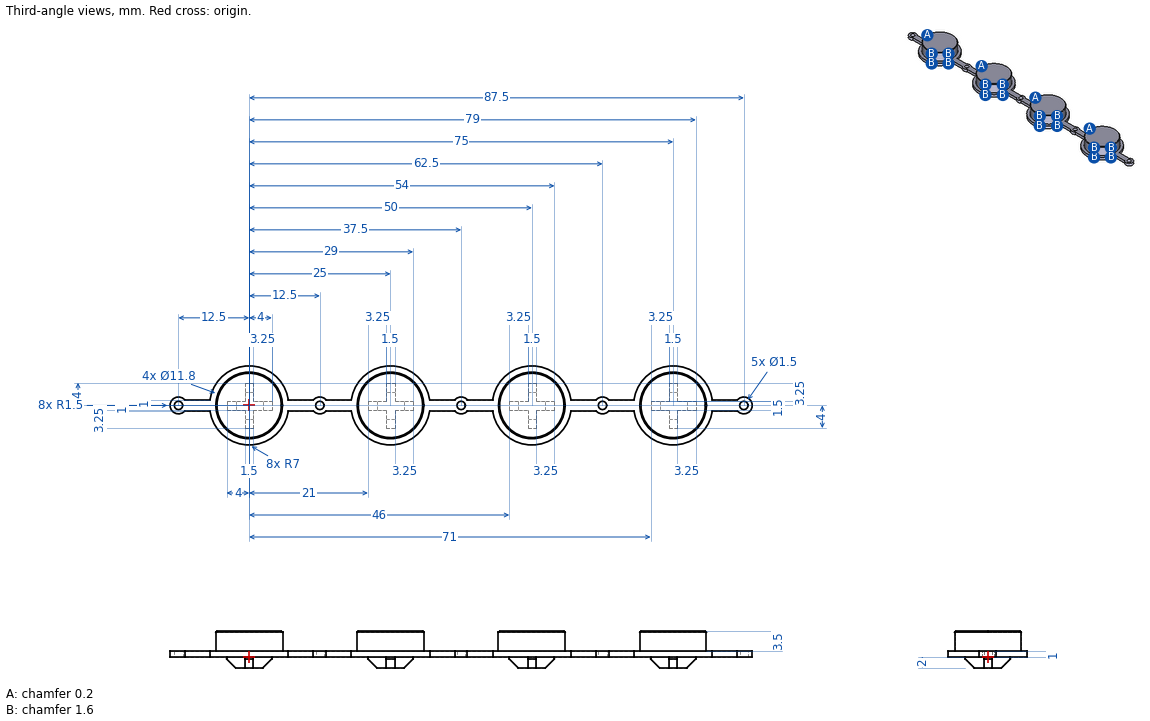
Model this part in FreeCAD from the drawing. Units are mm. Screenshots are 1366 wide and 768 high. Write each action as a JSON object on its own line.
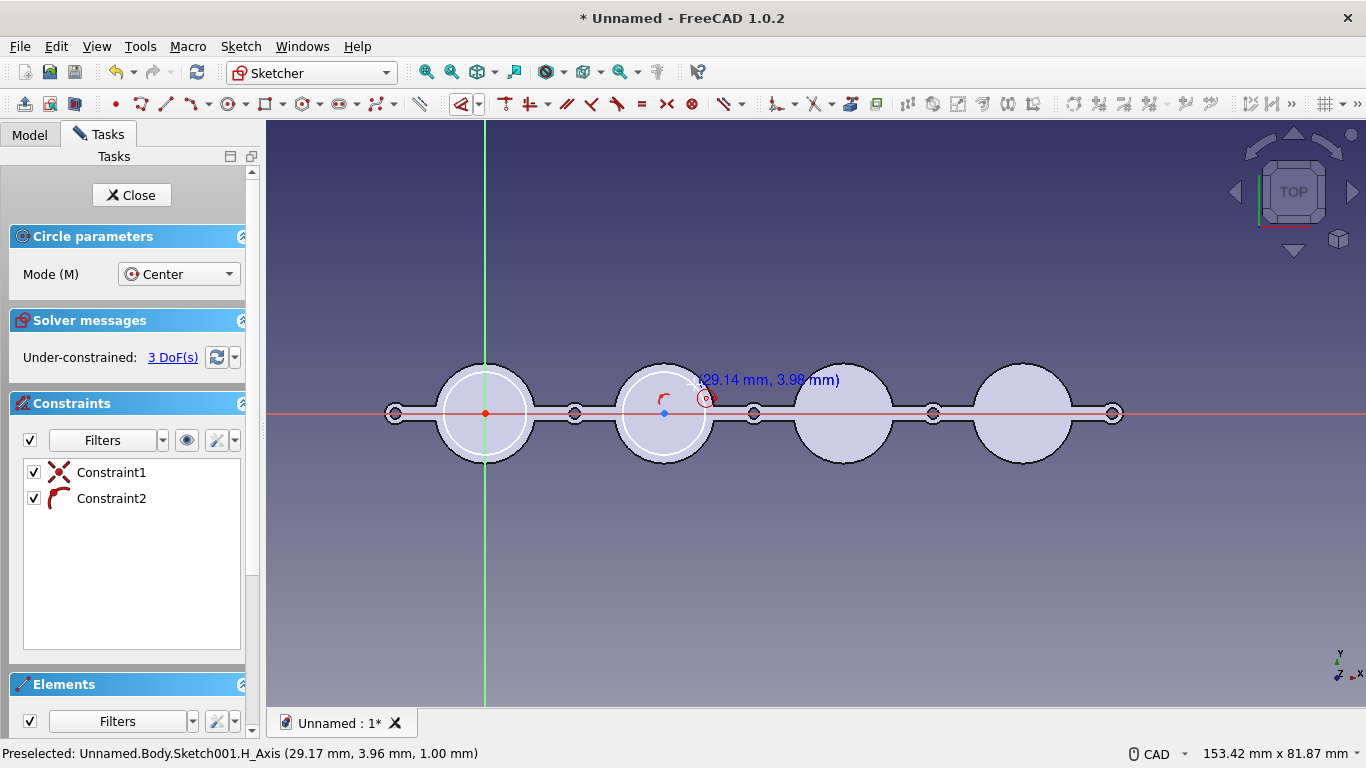
{"action": "left_click", "coordinate": [844, 414]}
{"action": "left_click", "coordinate": [873, 384]}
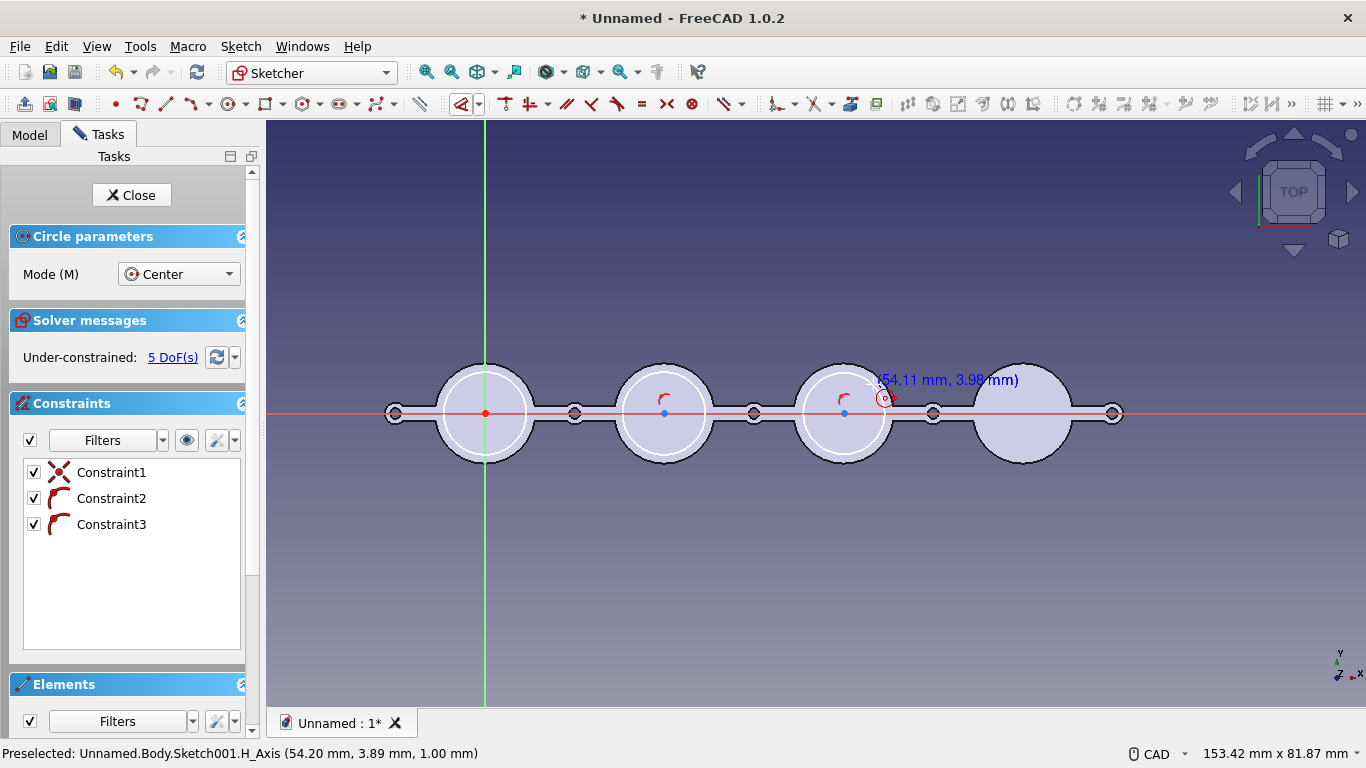
{"action": "left_click", "coordinate": [1023, 414]}
{"action": "left_click", "coordinate": [1053, 384]}
{"action": "key", "text": "Escape"}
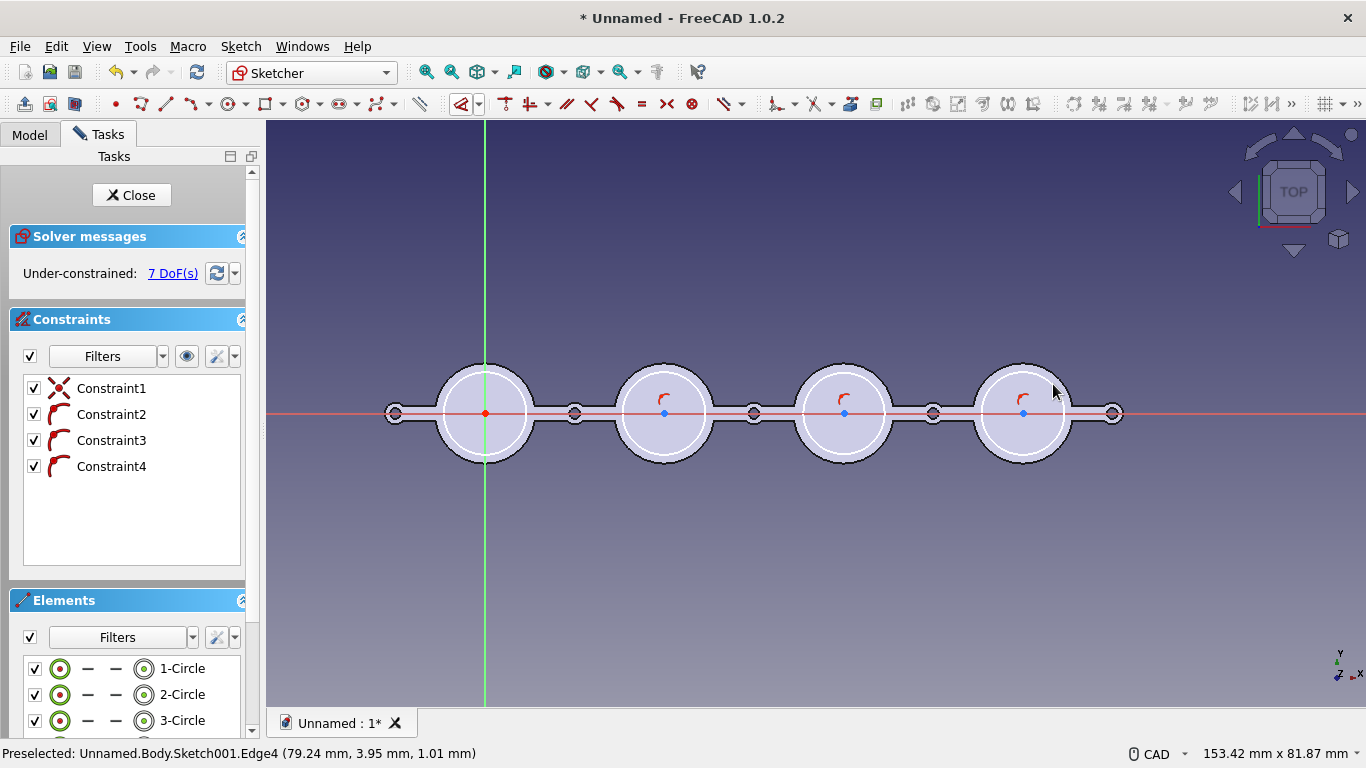
{"action": "left_click", "coordinate": [514, 384]}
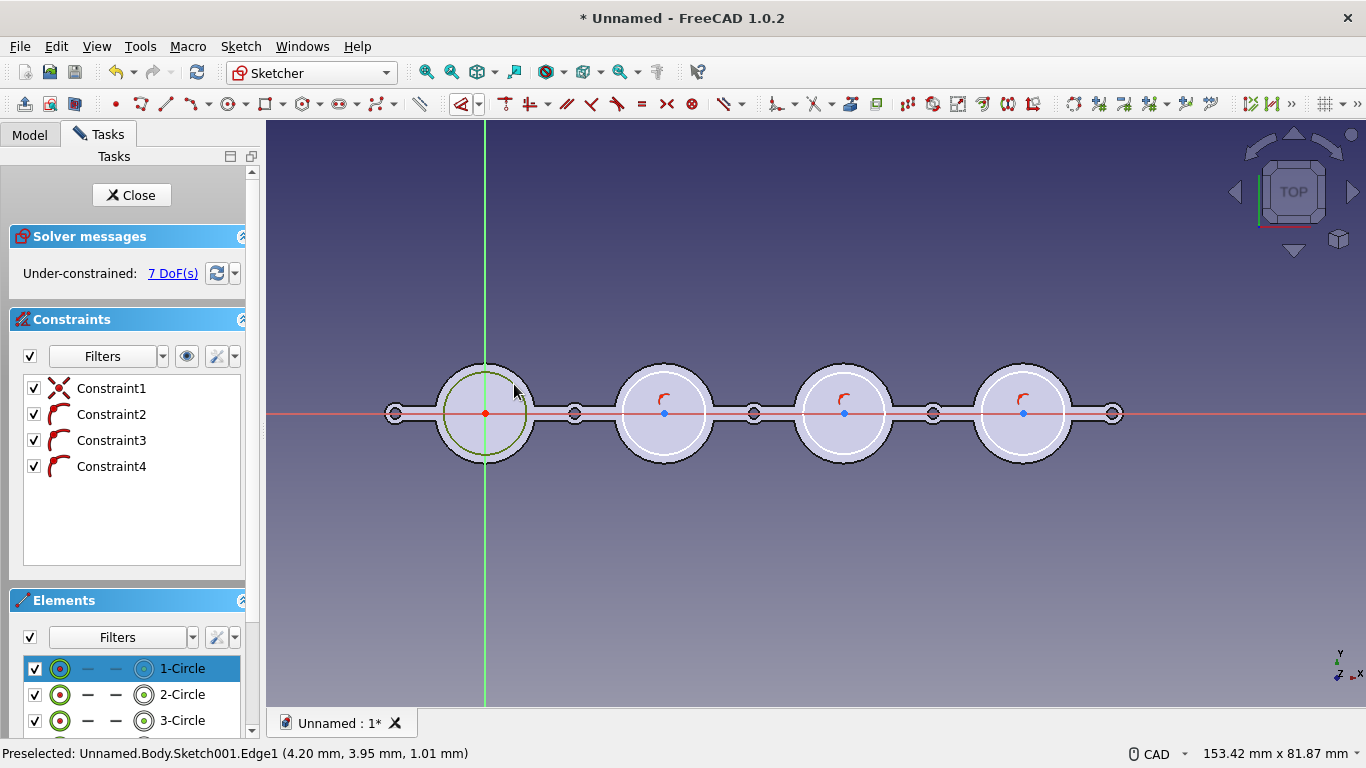
{"action": "left_click", "coordinate": [693, 384]}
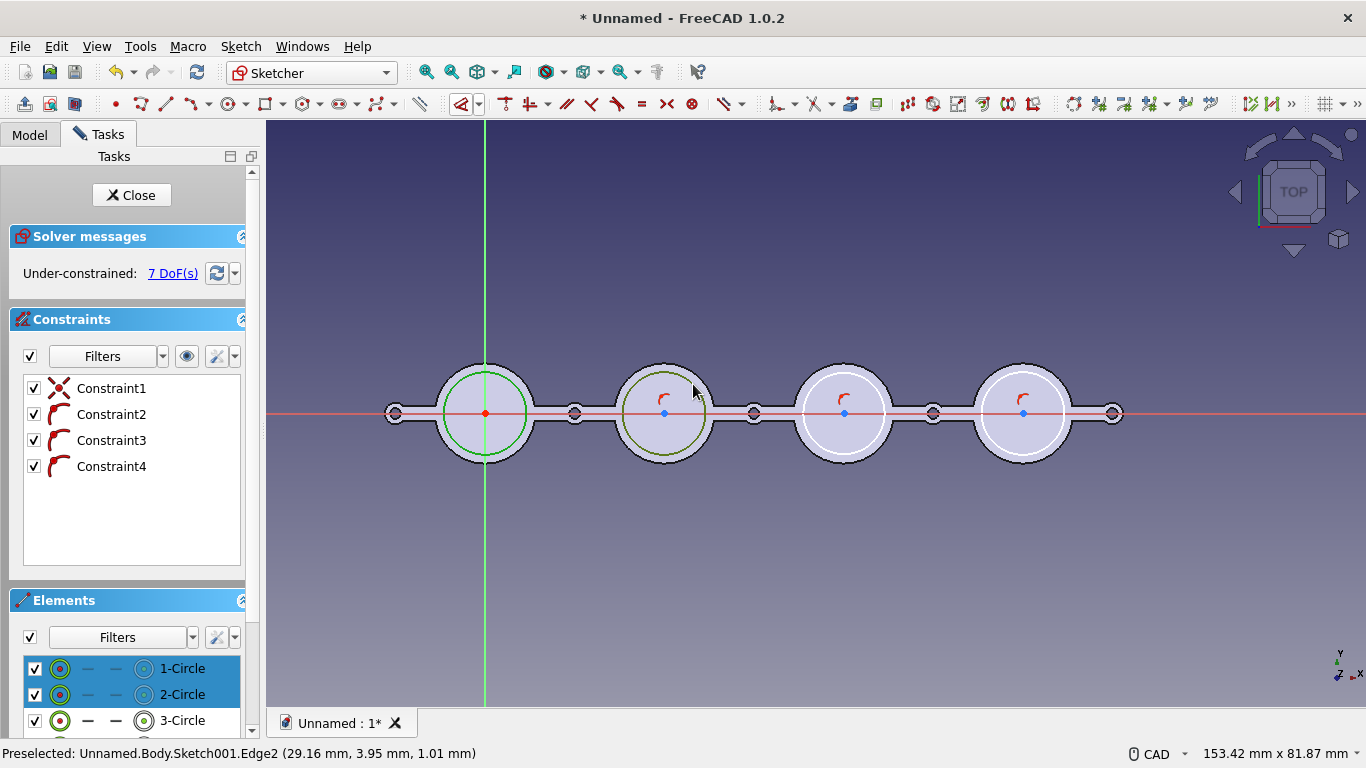
{"action": "left_click", "coordinate": [873, 385]}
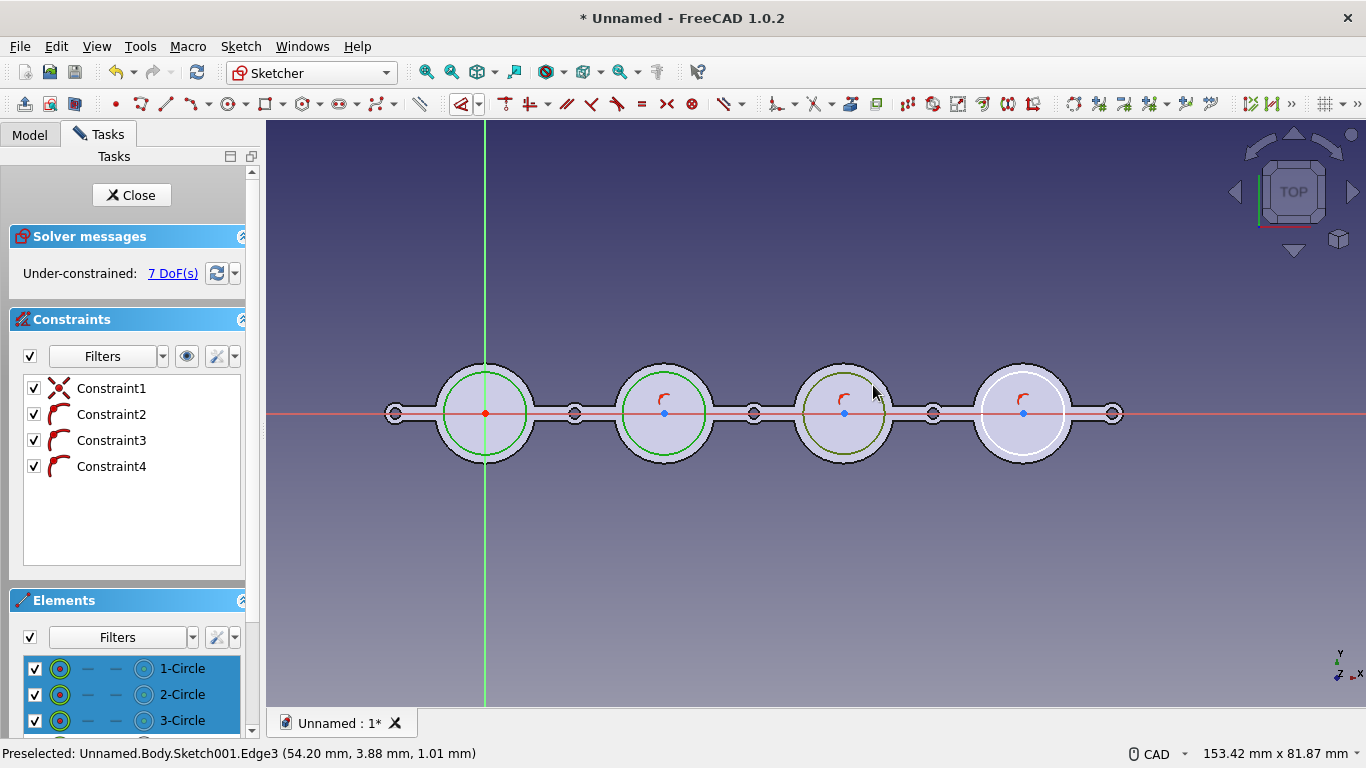
{"action": "left_click", "coordinate": [1052, 384]}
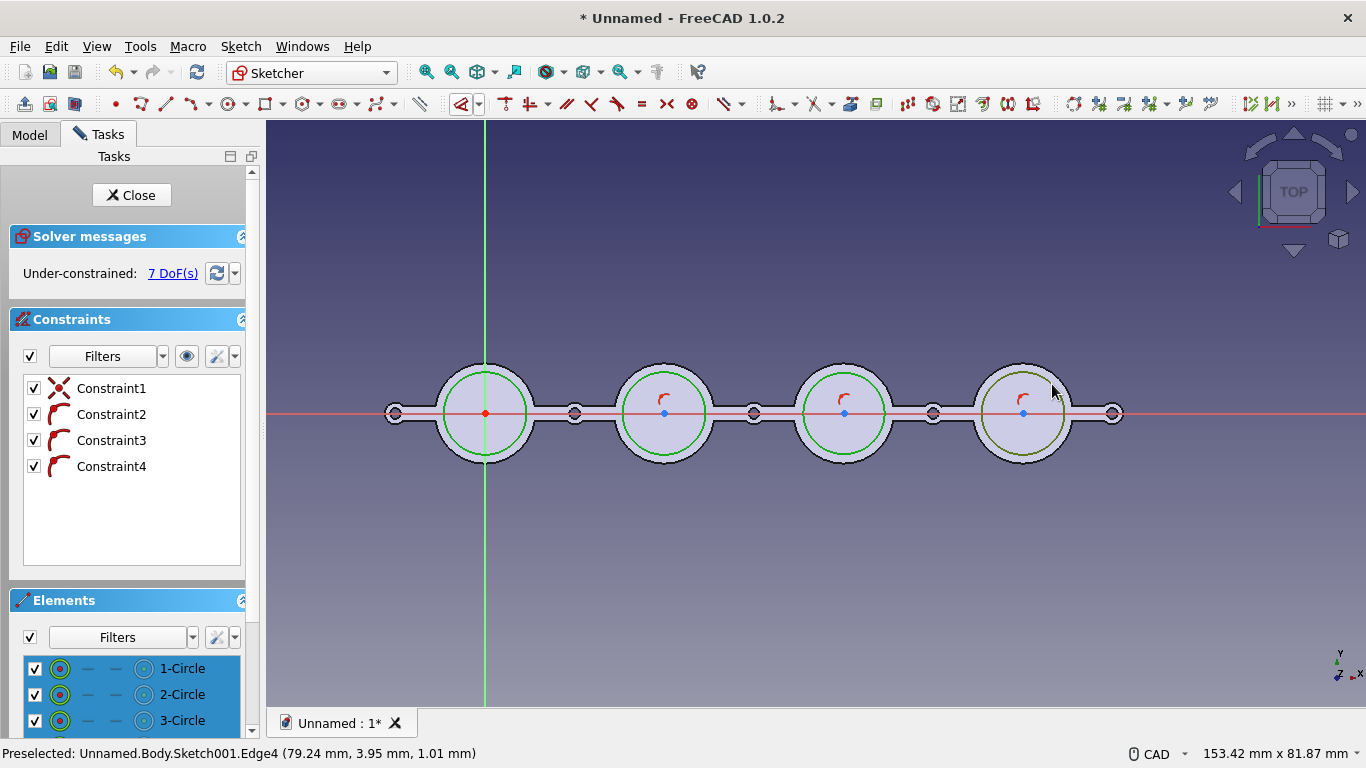
{"action": "key", "text": "e"}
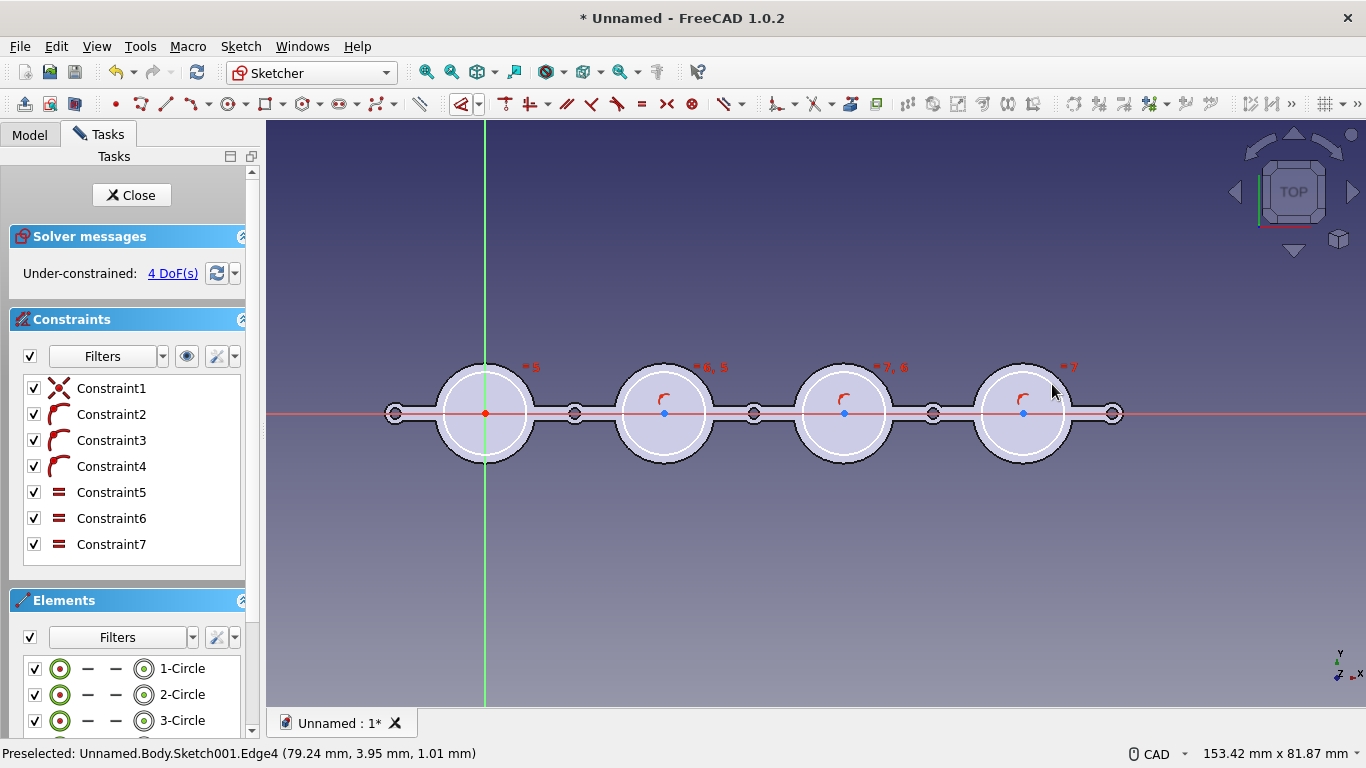
{"action": "left_click", "coordinate": [514, 384]}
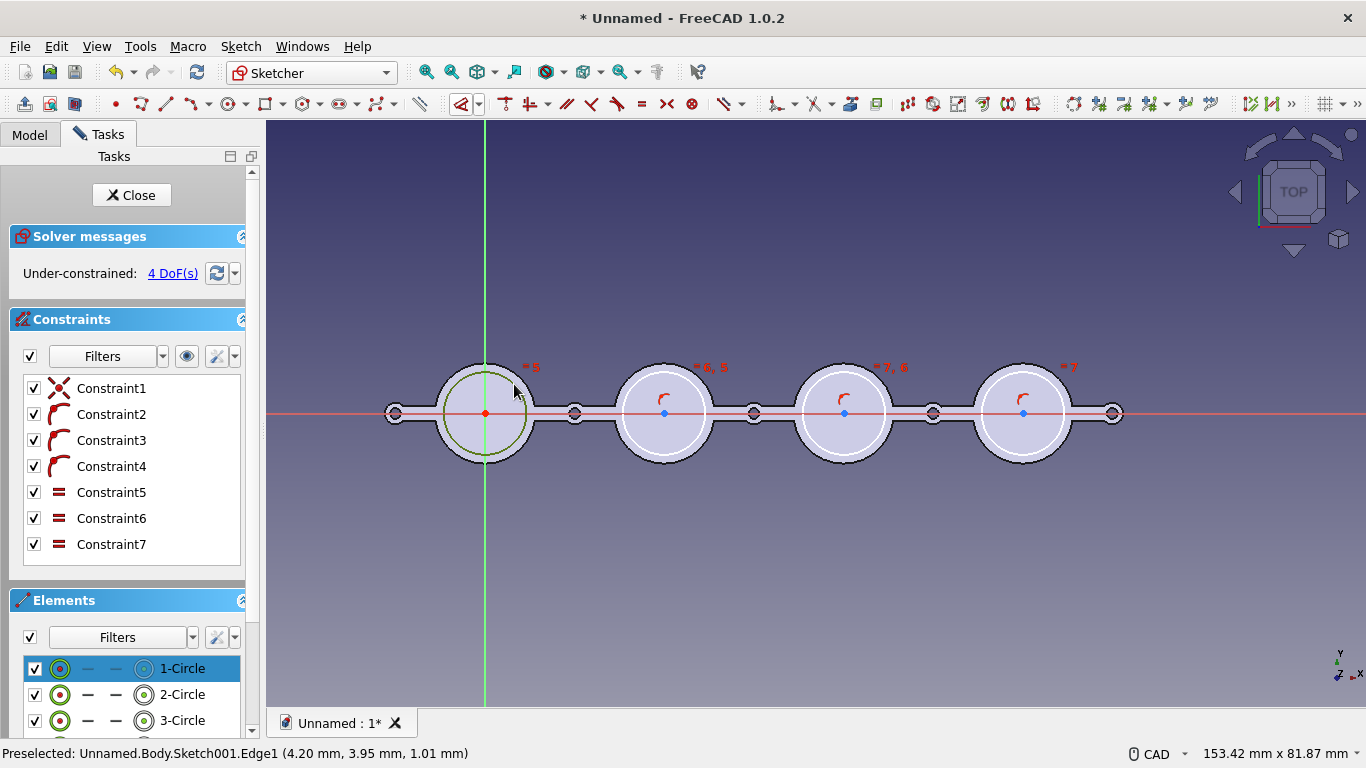
{"action": "key", "text": "k o"}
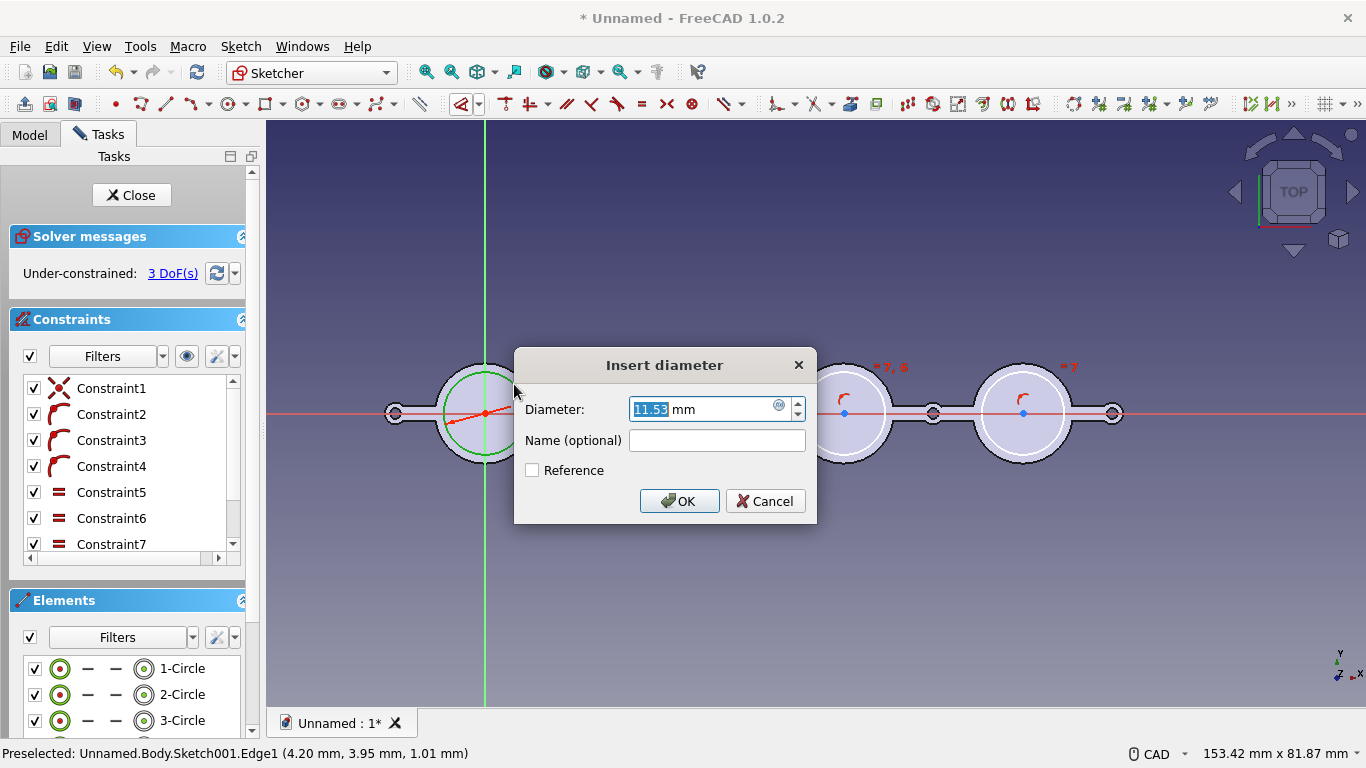
{"action": "type", "text": "11.8"}
{"action": "key", "text": "Return"}